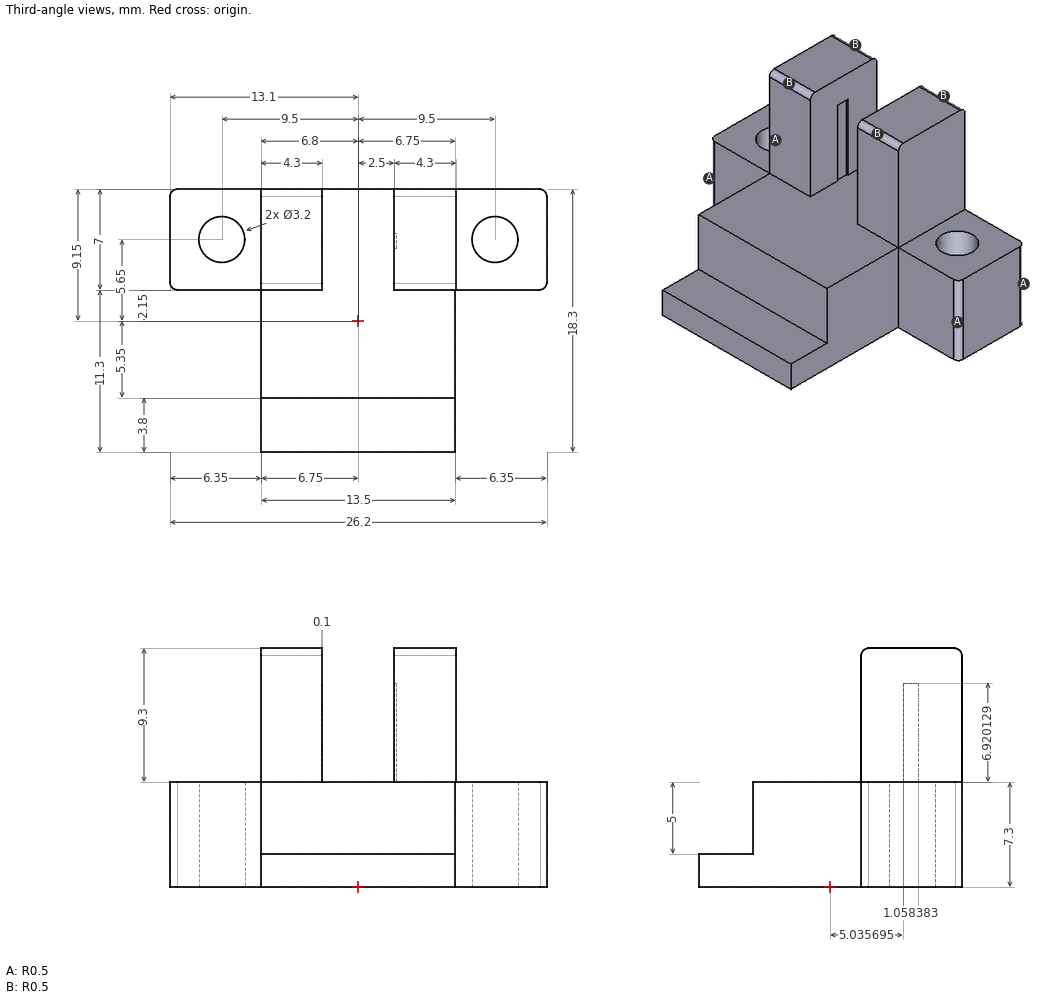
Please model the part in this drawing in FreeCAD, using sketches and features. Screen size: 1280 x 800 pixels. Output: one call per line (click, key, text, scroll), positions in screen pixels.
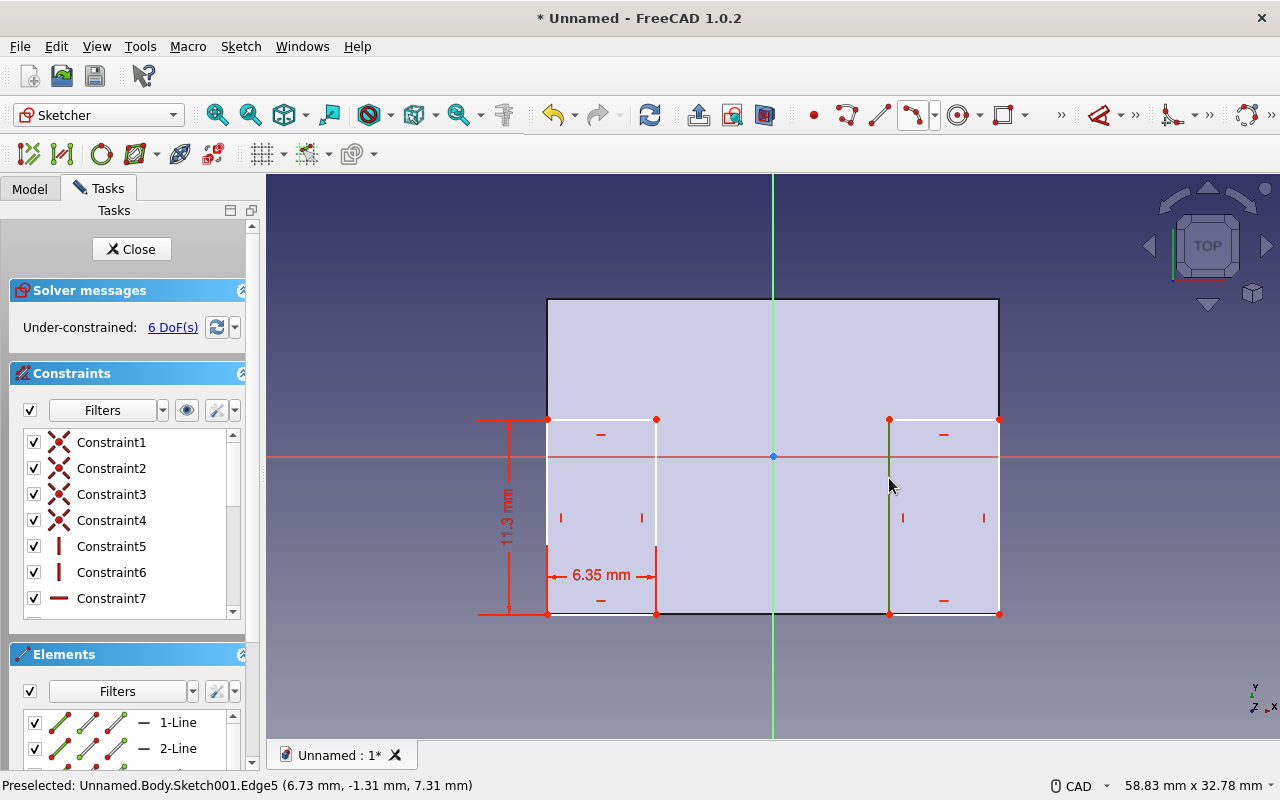
key(i)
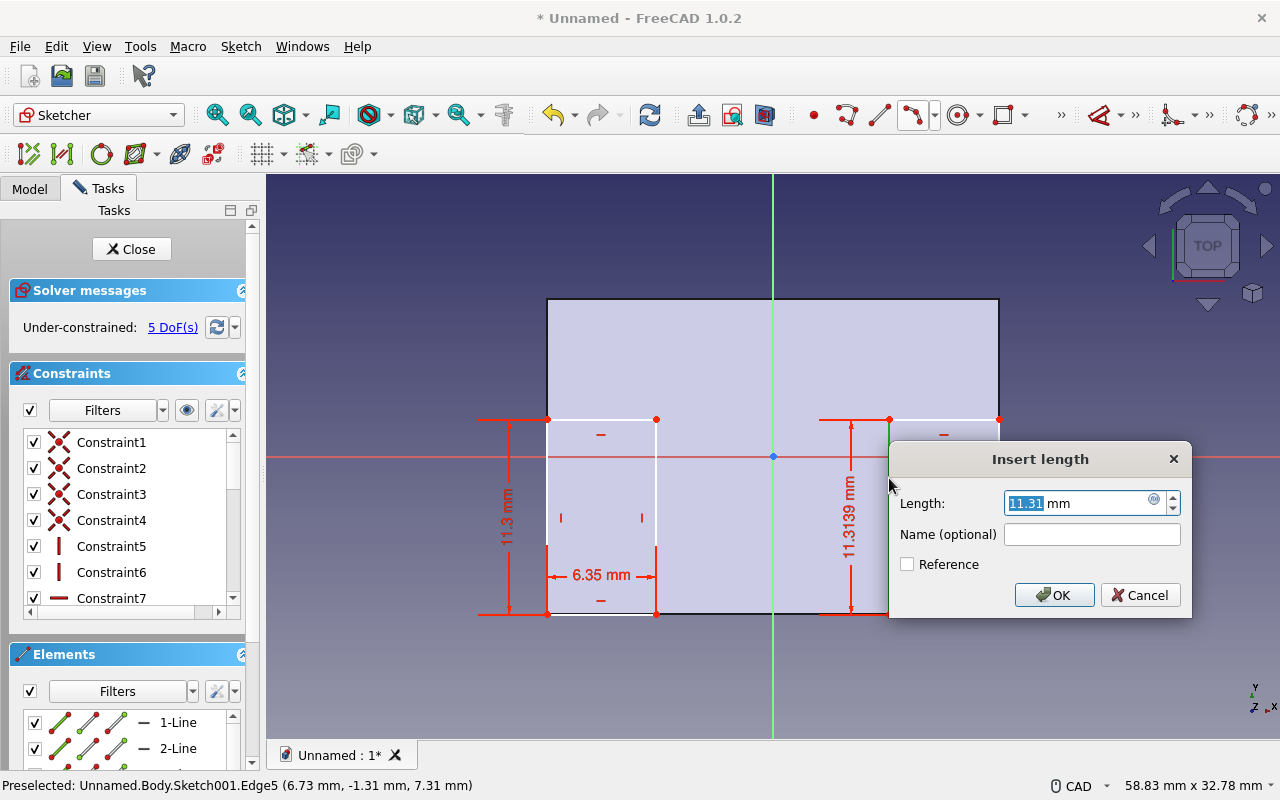
text(11.3)
key(Return)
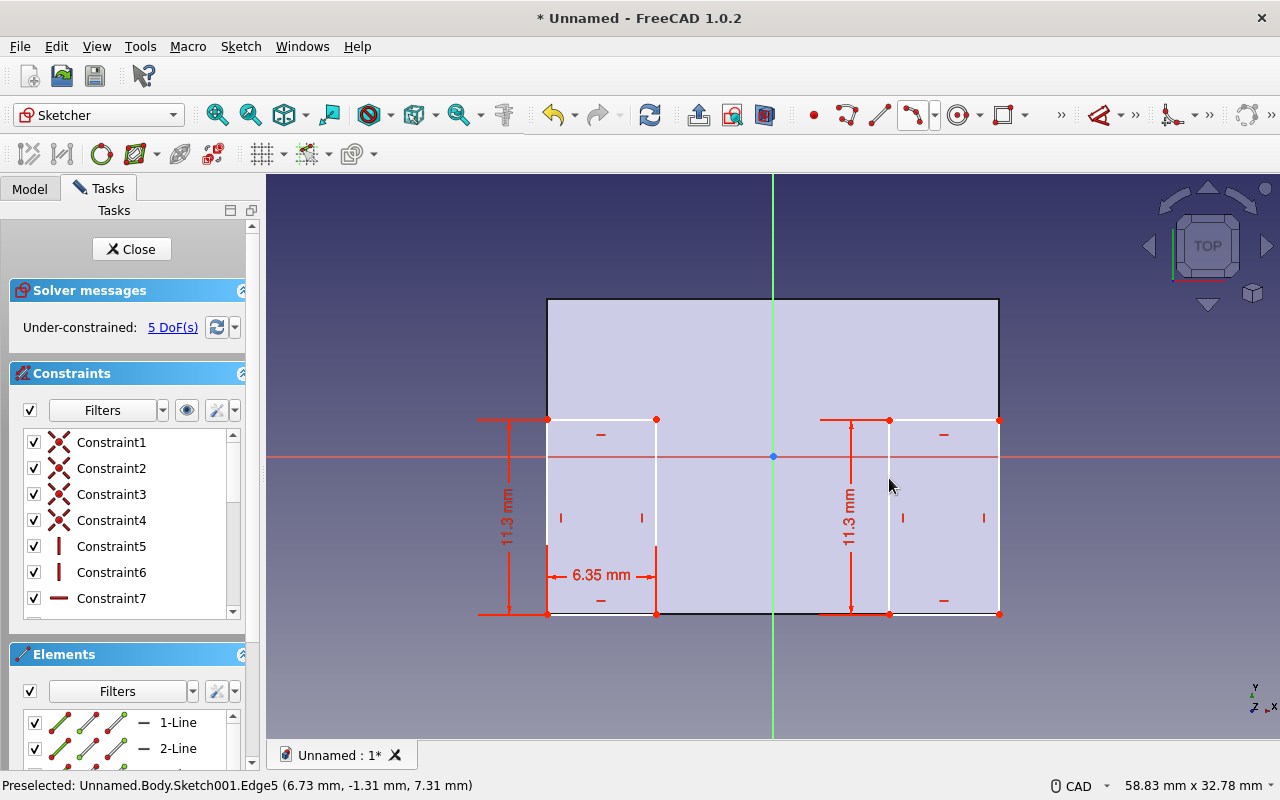
click(922, 615)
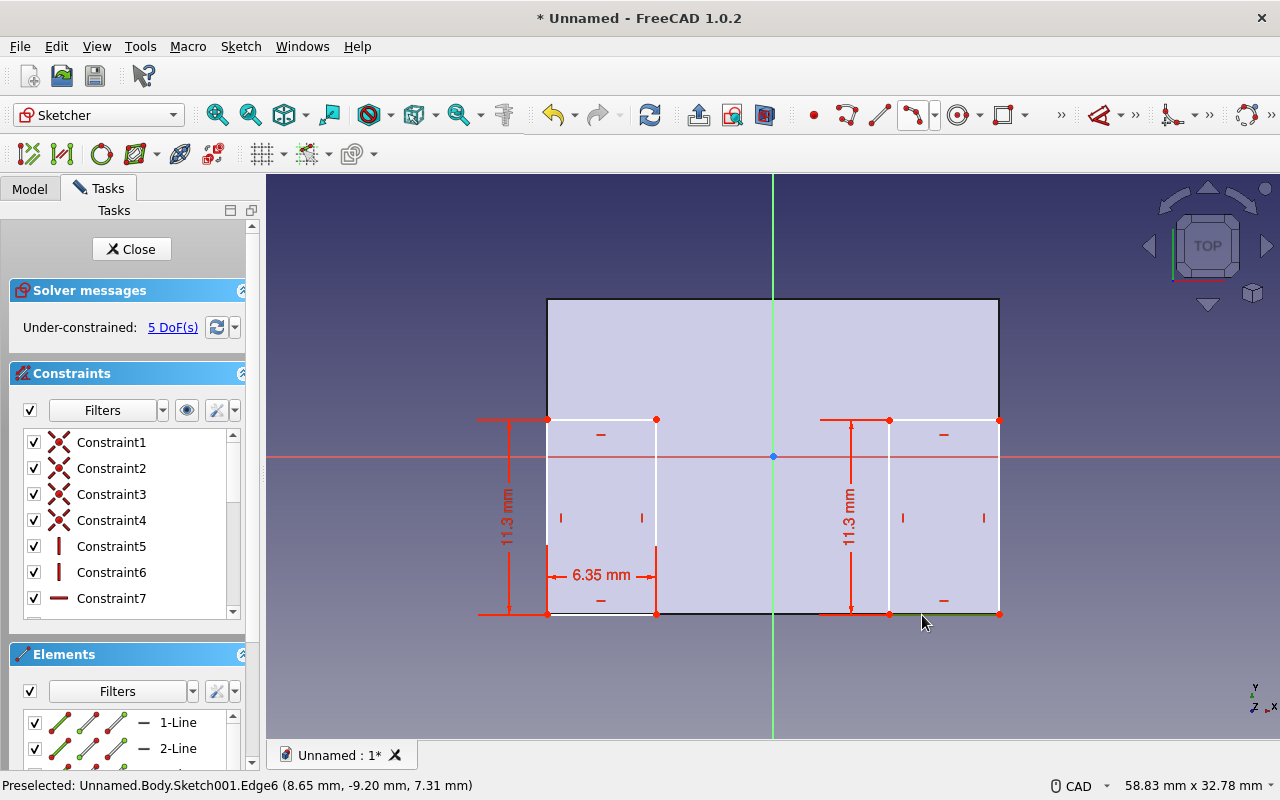
key(l)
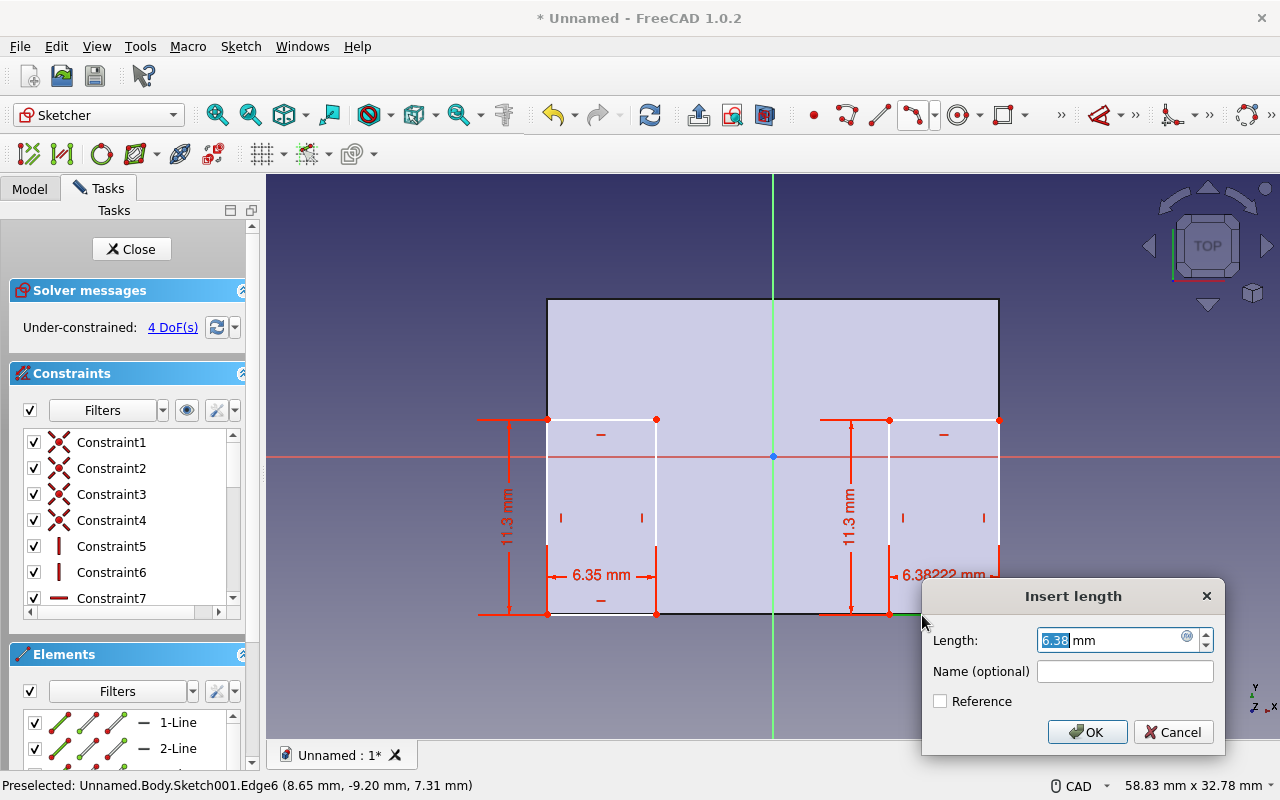
text(6.35)
key(Return)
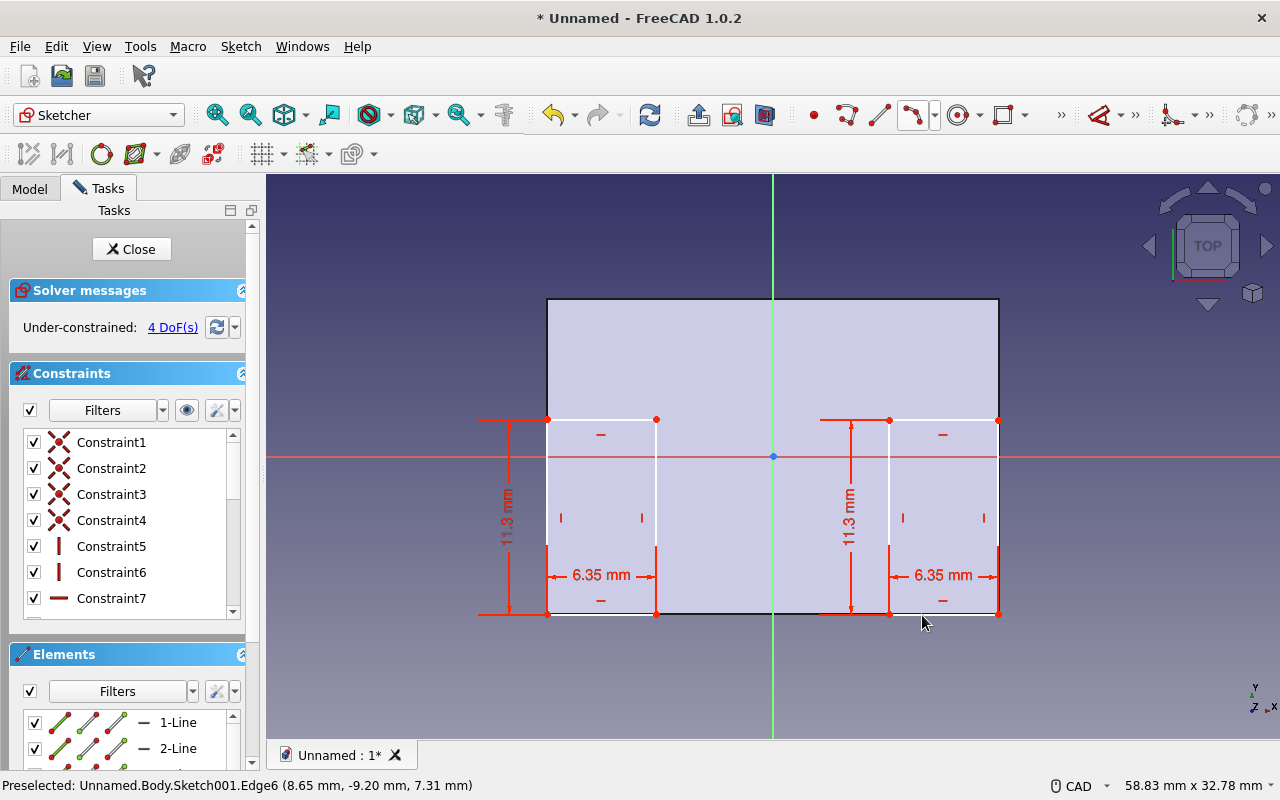
click(547, 420)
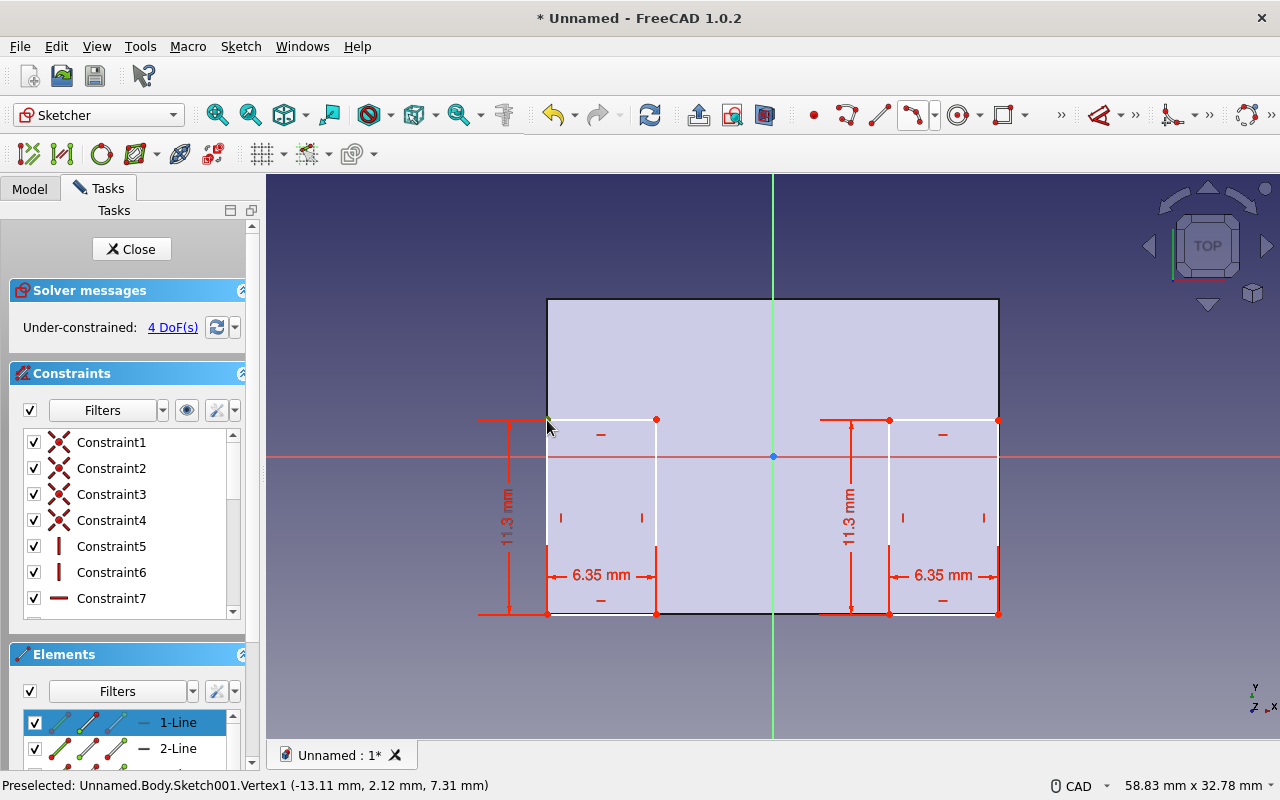
key(l)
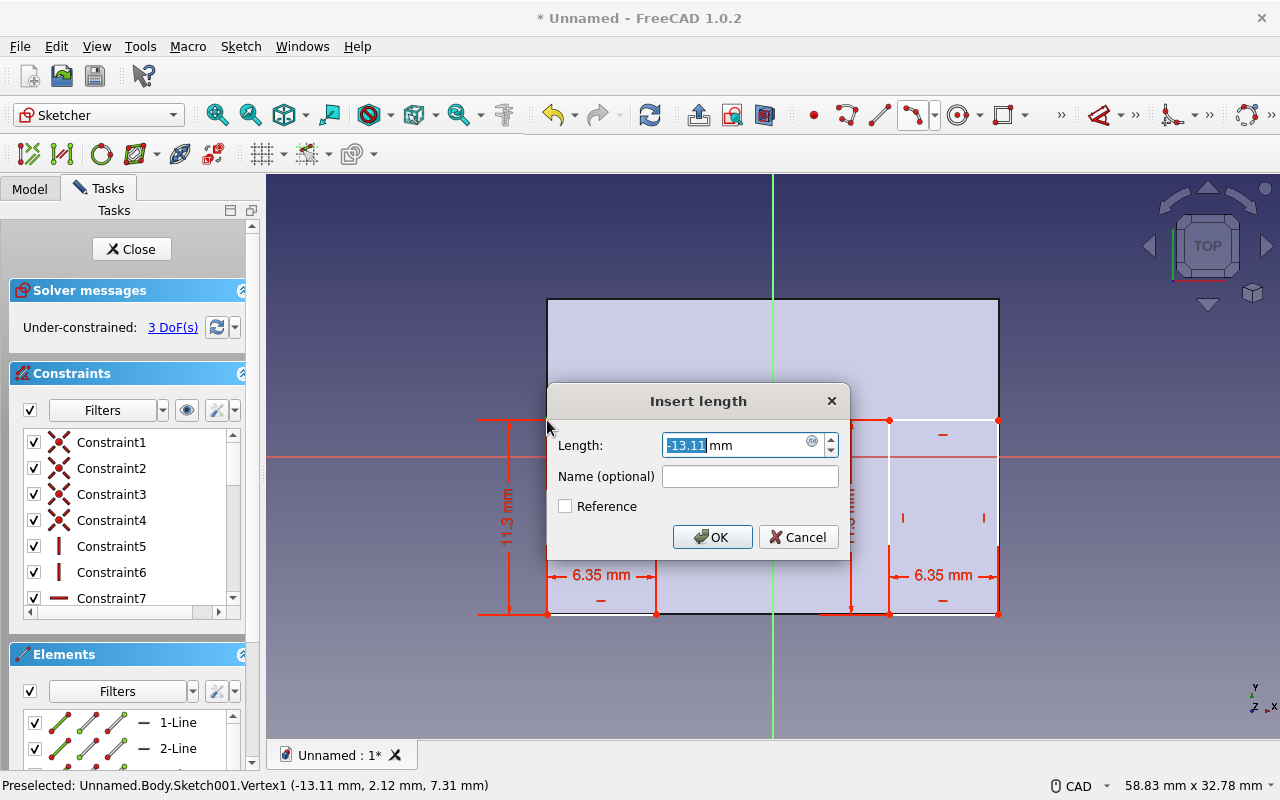
text(-13.1)
key(Return)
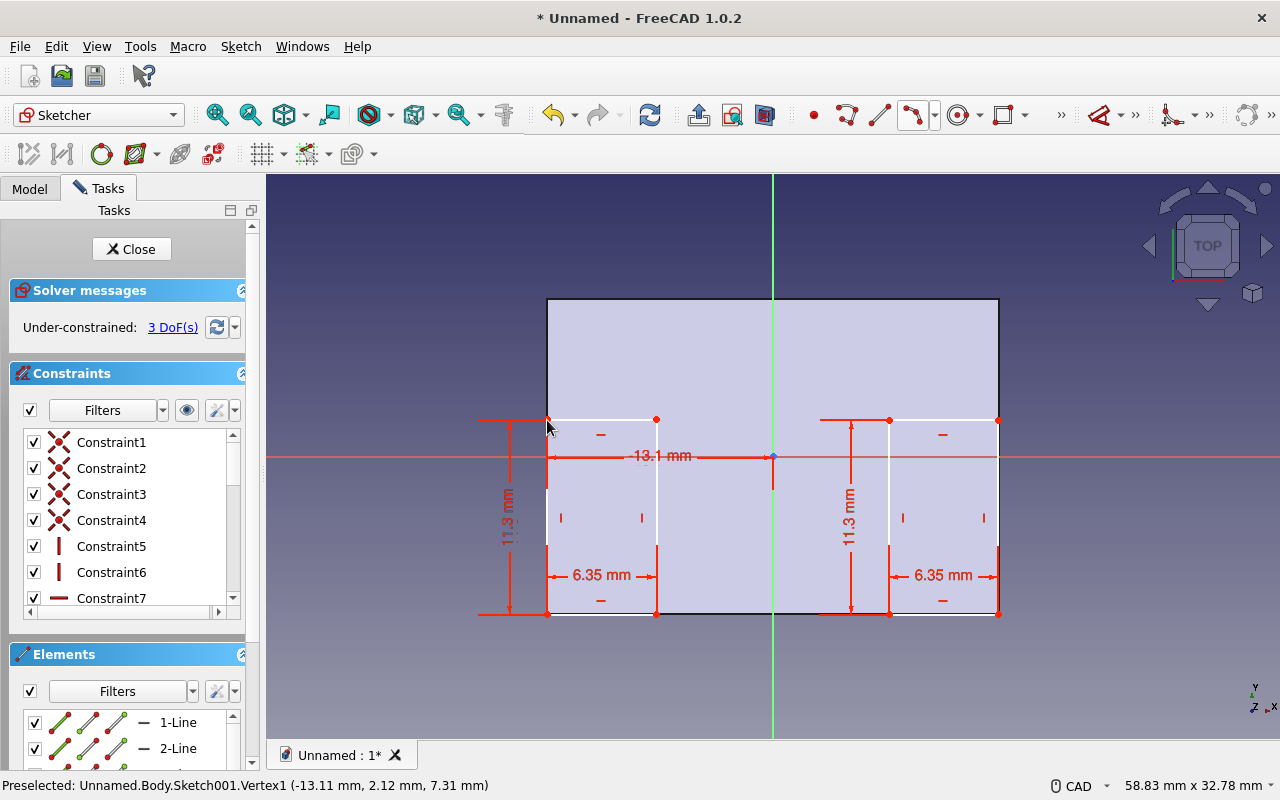
click(547, 420)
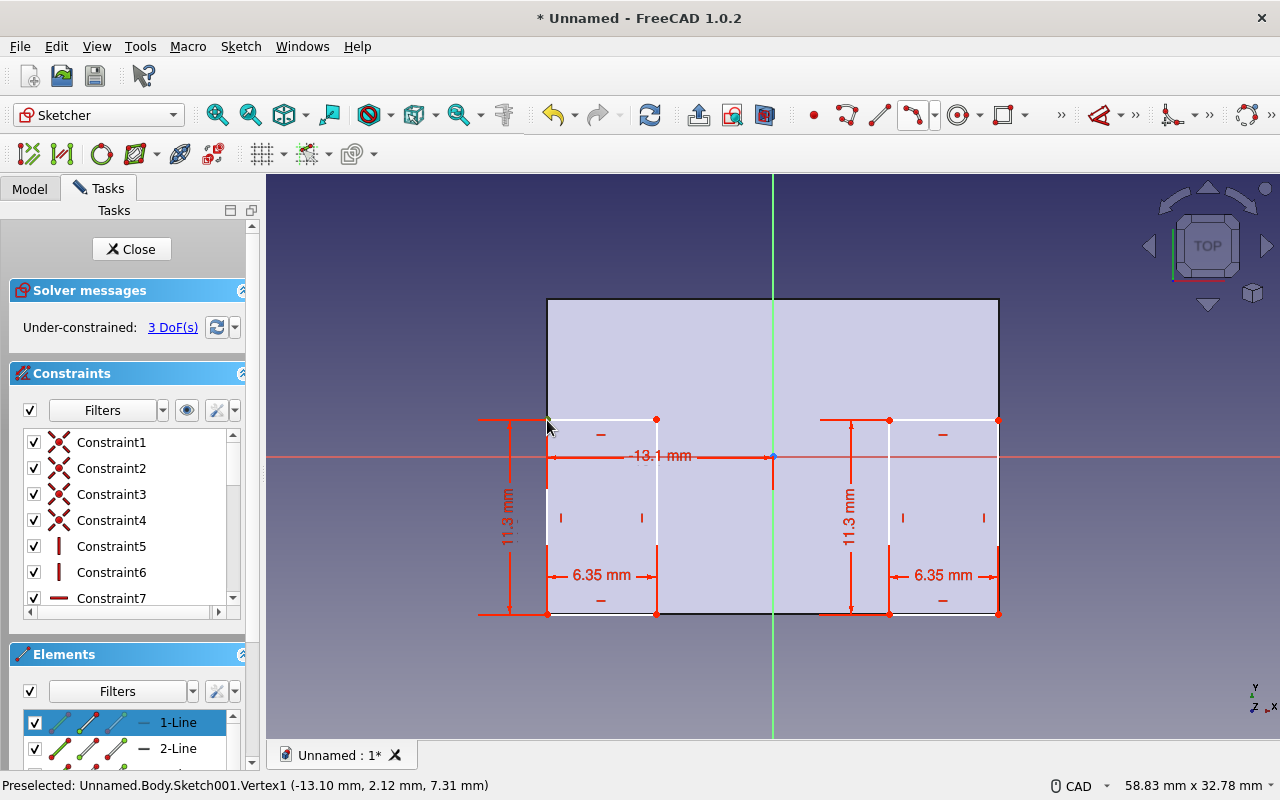
key(i)